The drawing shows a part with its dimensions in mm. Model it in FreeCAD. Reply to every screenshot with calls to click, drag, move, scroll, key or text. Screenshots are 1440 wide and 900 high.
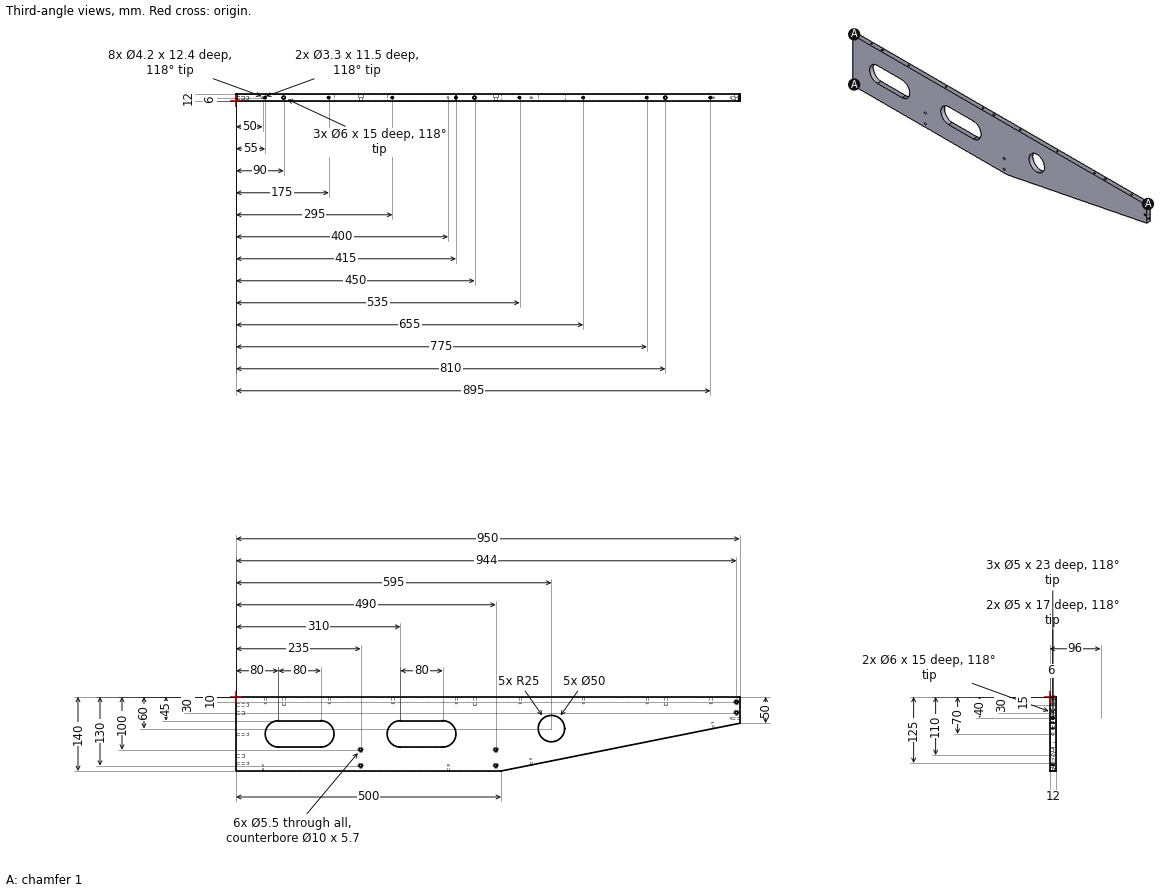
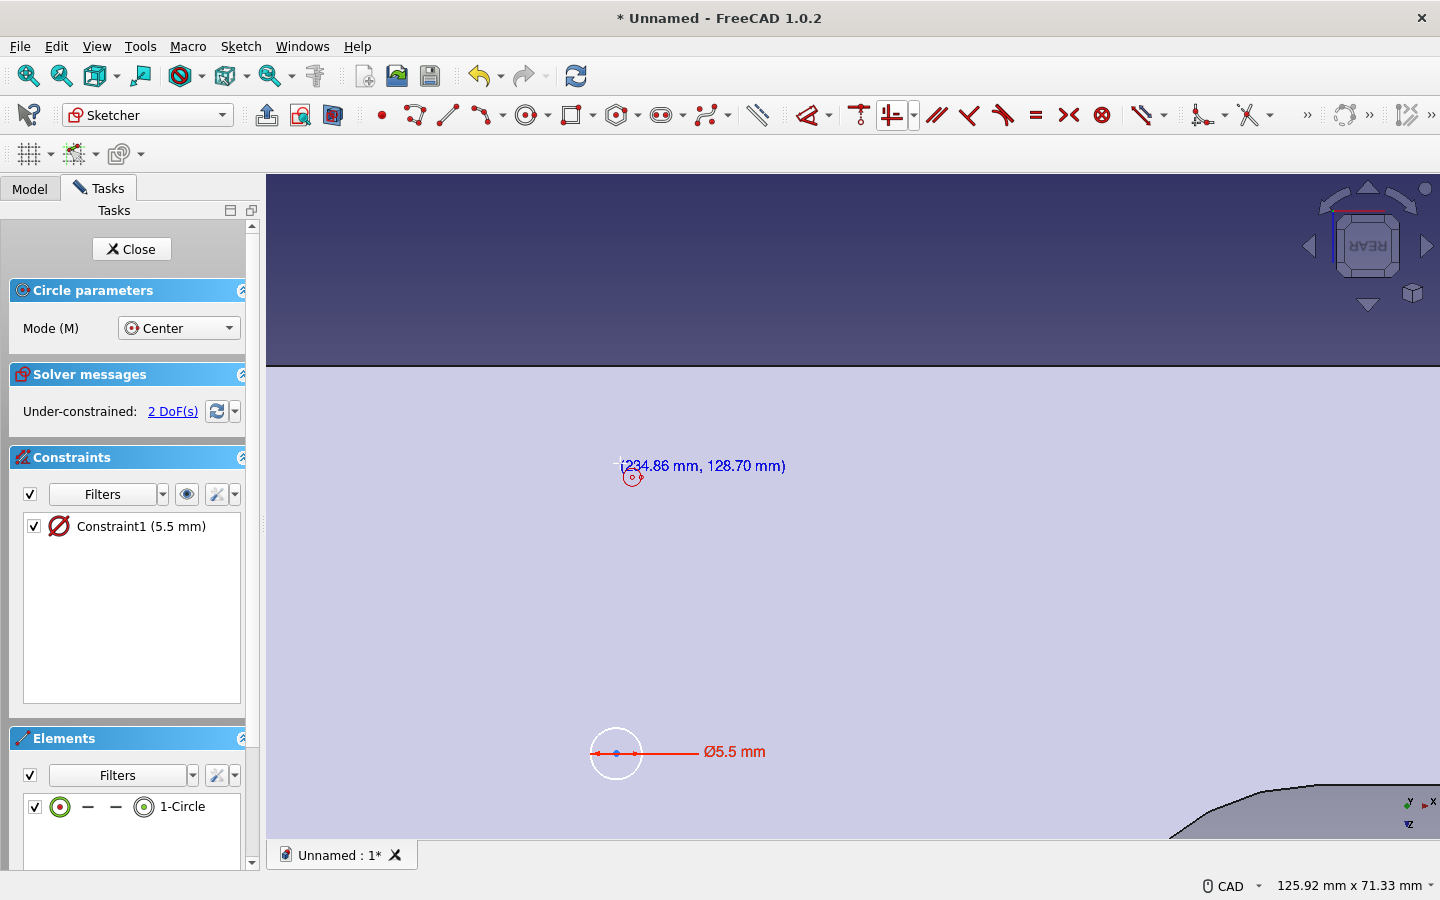
scroll(620, 463, down, 13)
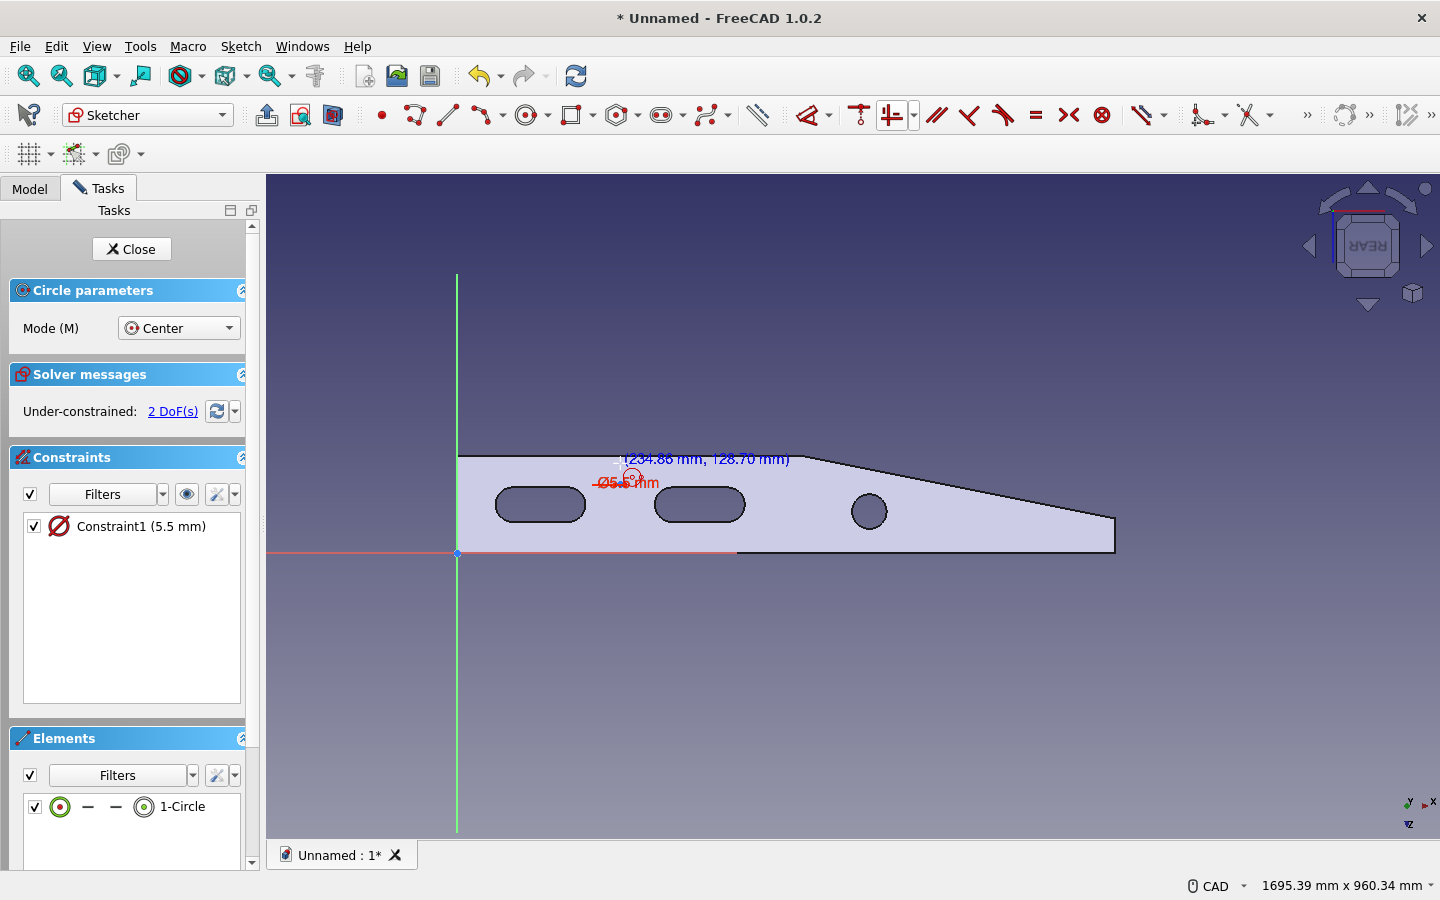
click(620, 463)
move(621, 462)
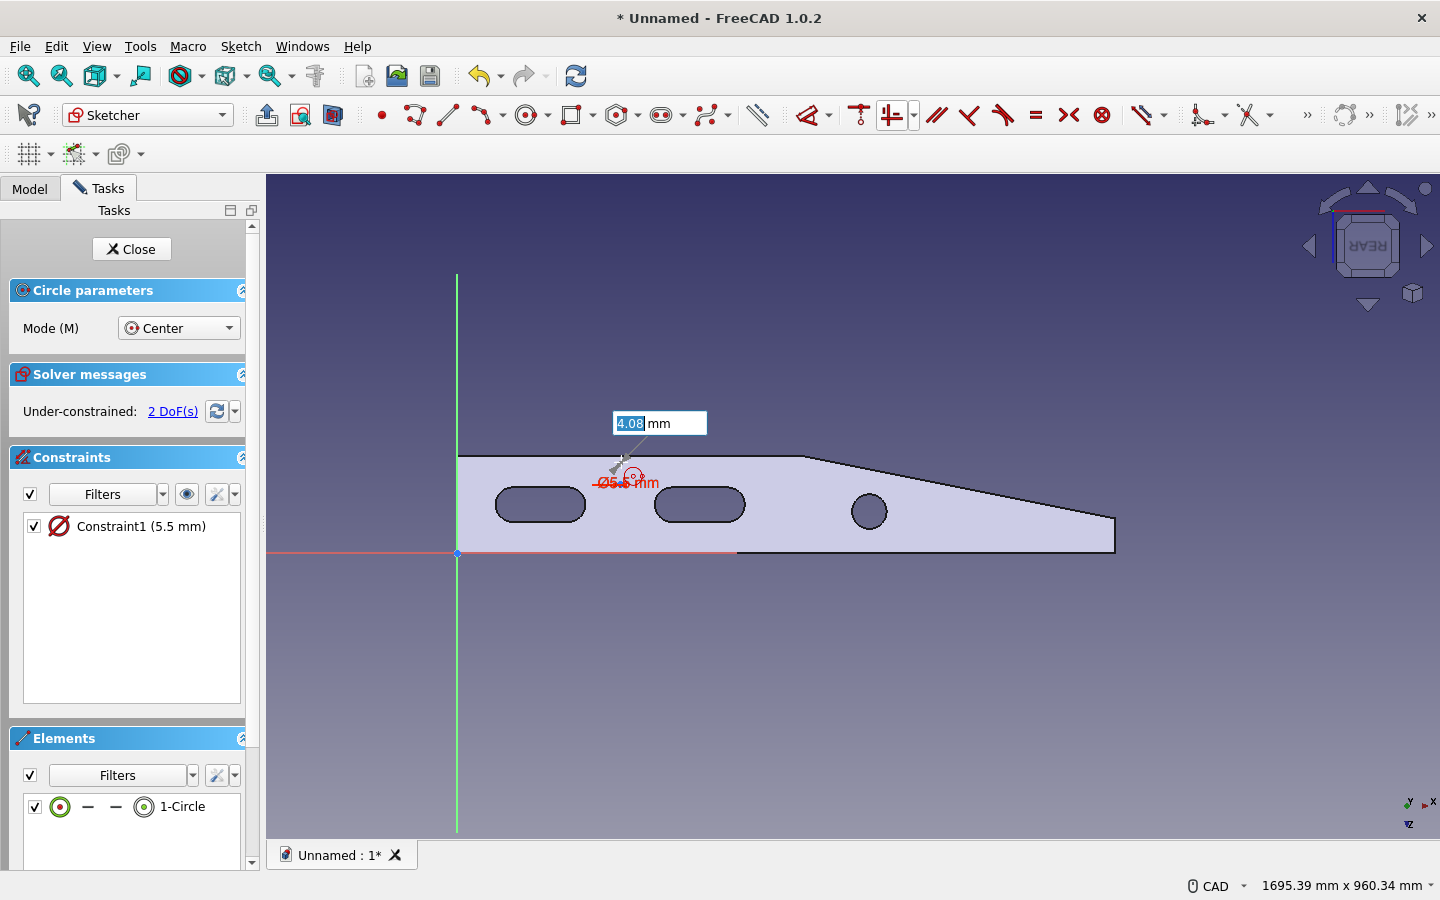
text(5.5)
key(Return)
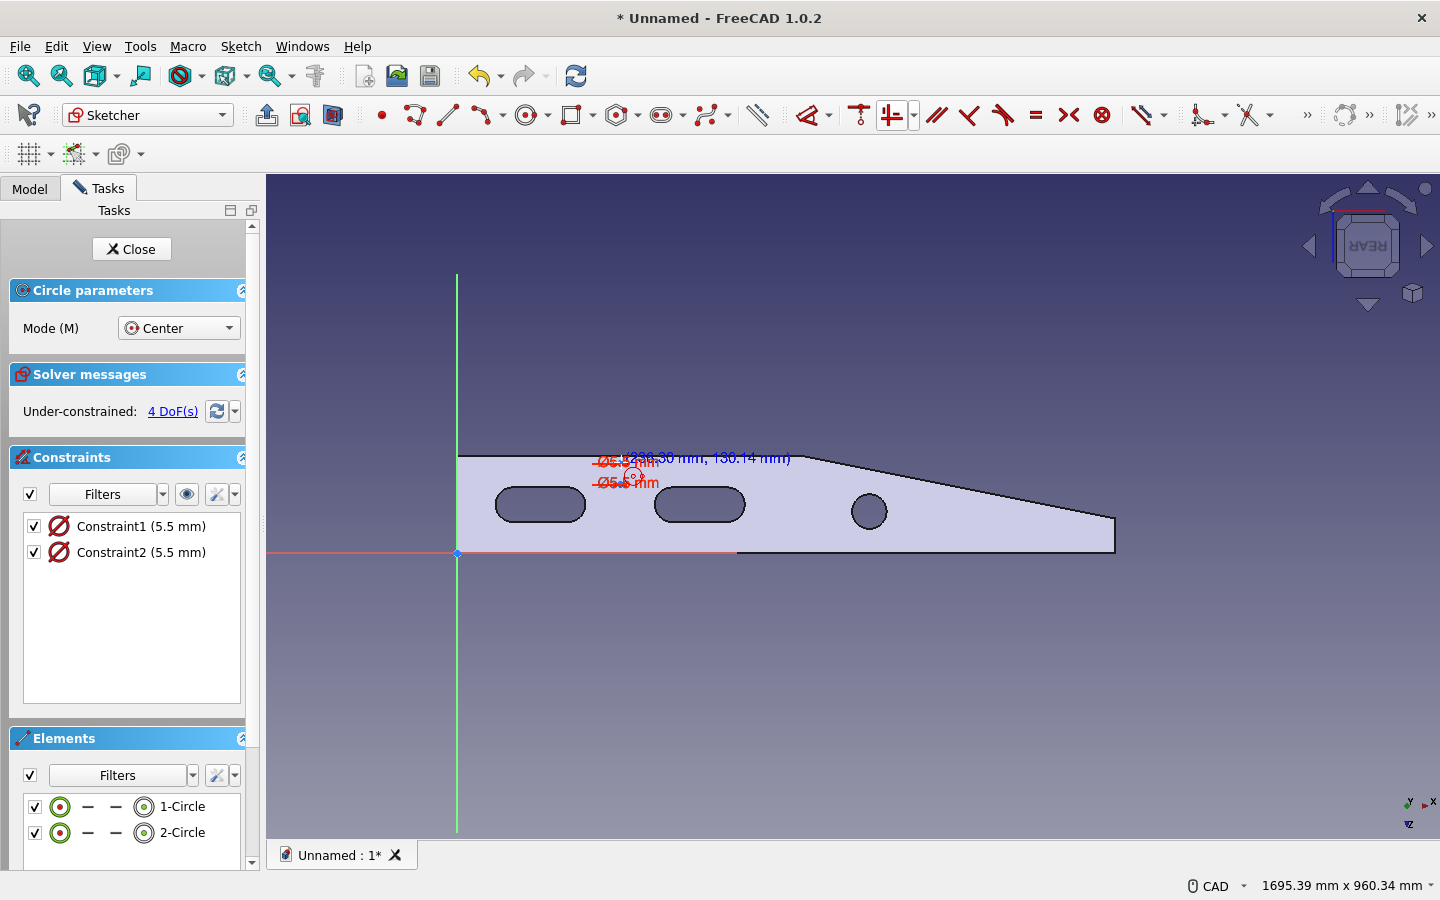
scroll(797, 484, up, 13)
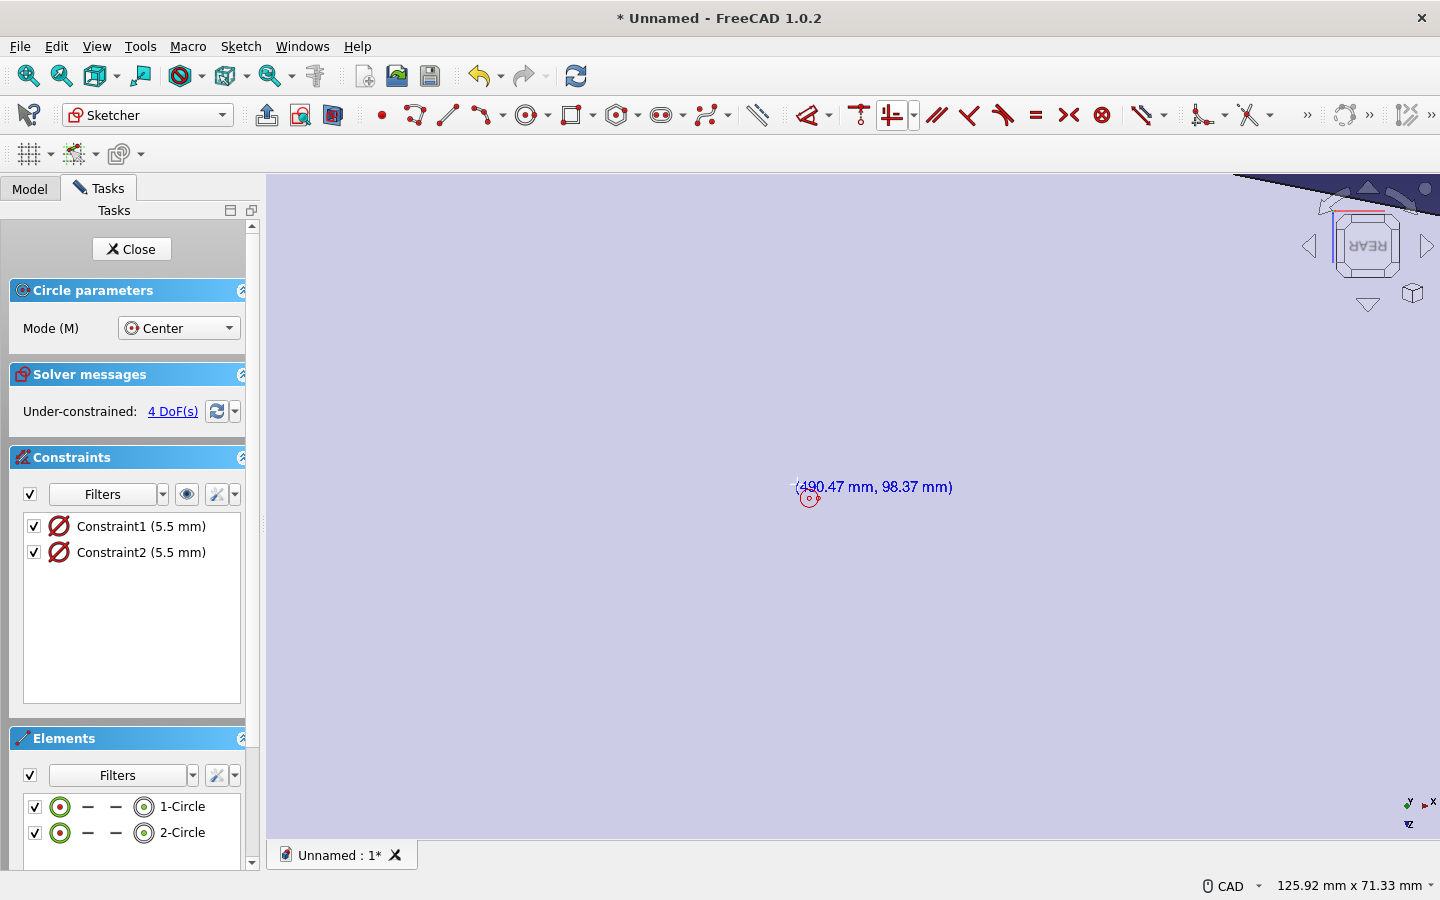
scroll(797, 484, down, 13)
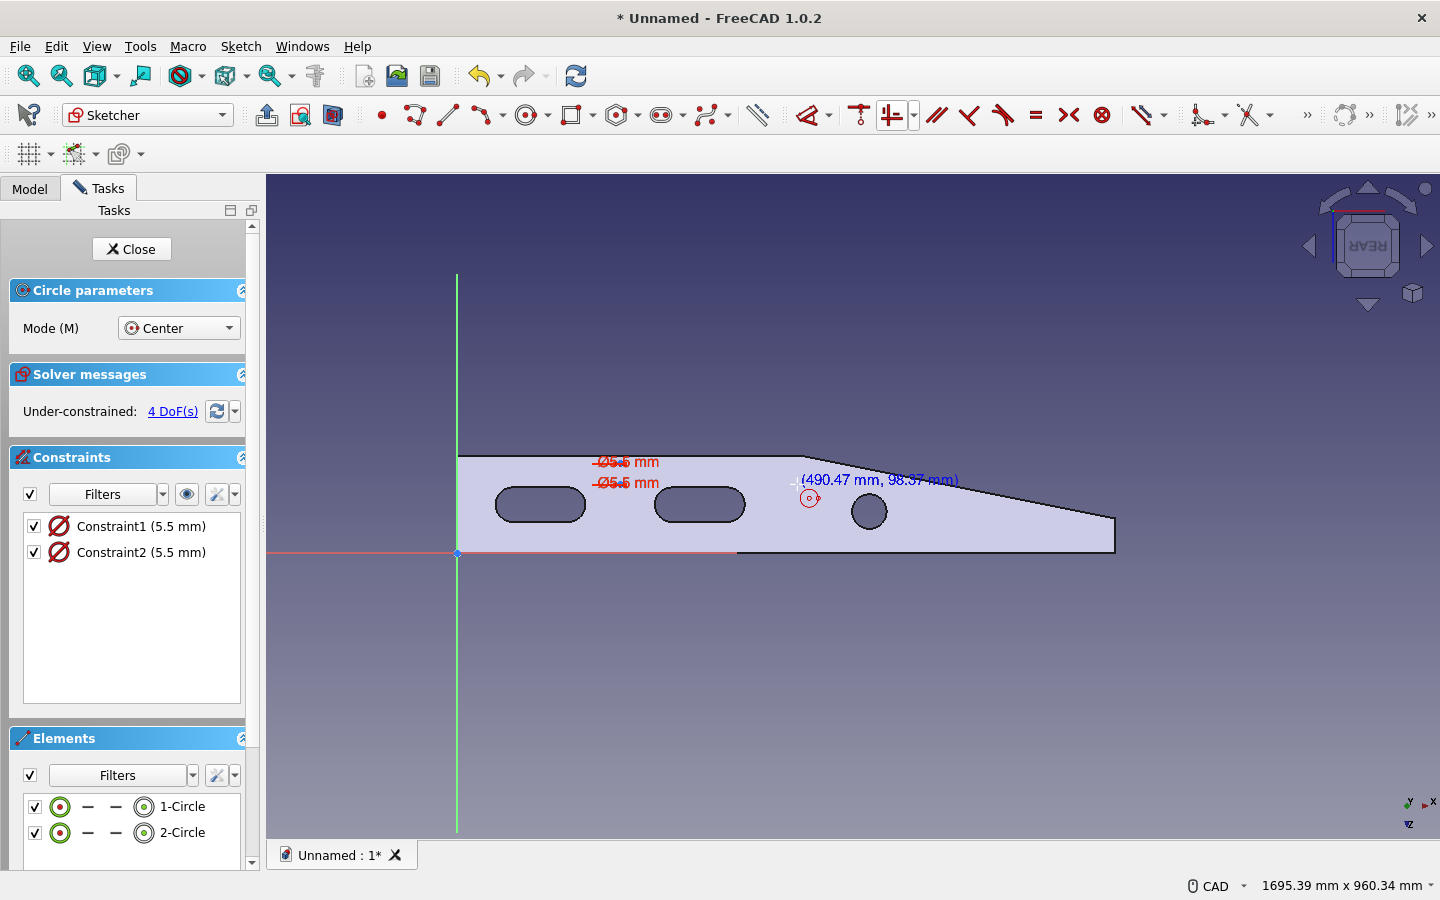
click(797, 484)
move(798, 483)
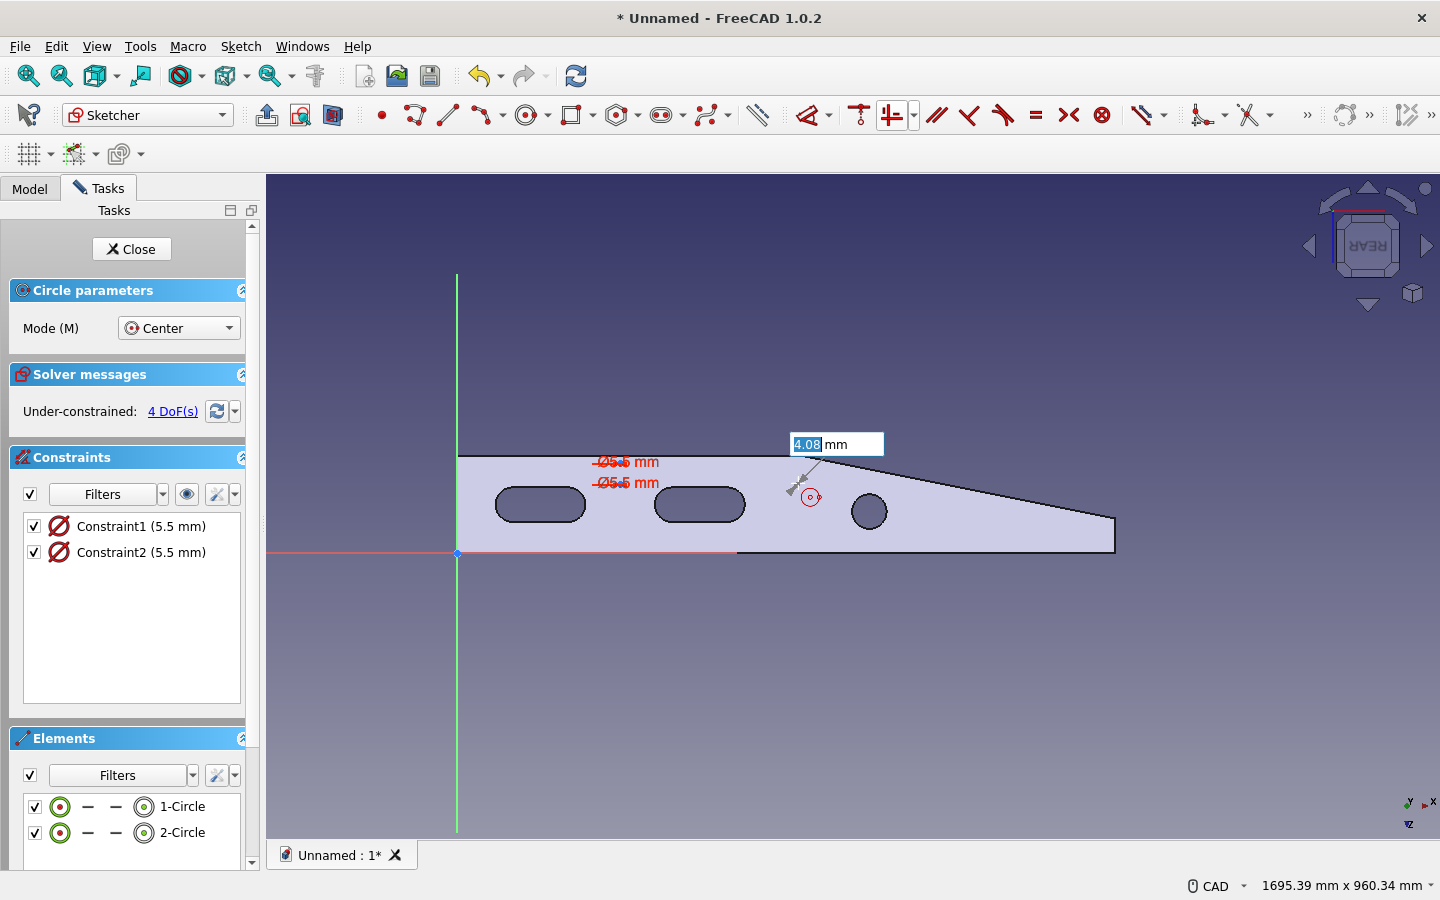
text(5.5)
key(Return)